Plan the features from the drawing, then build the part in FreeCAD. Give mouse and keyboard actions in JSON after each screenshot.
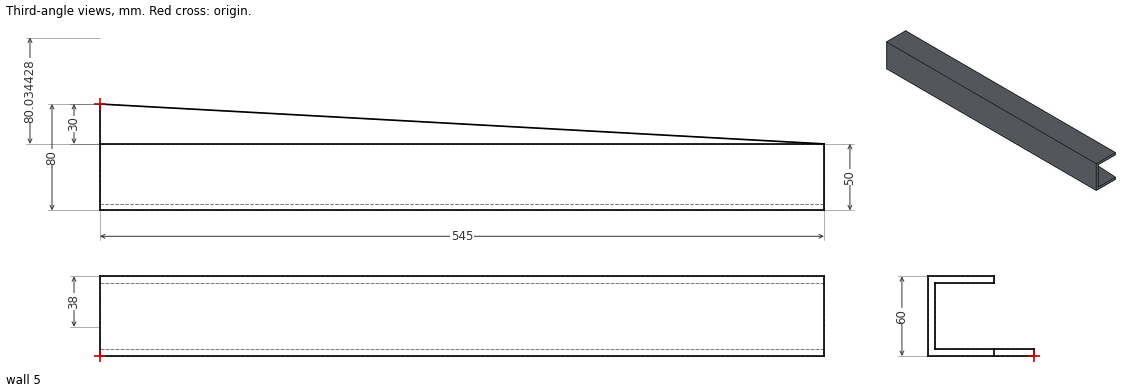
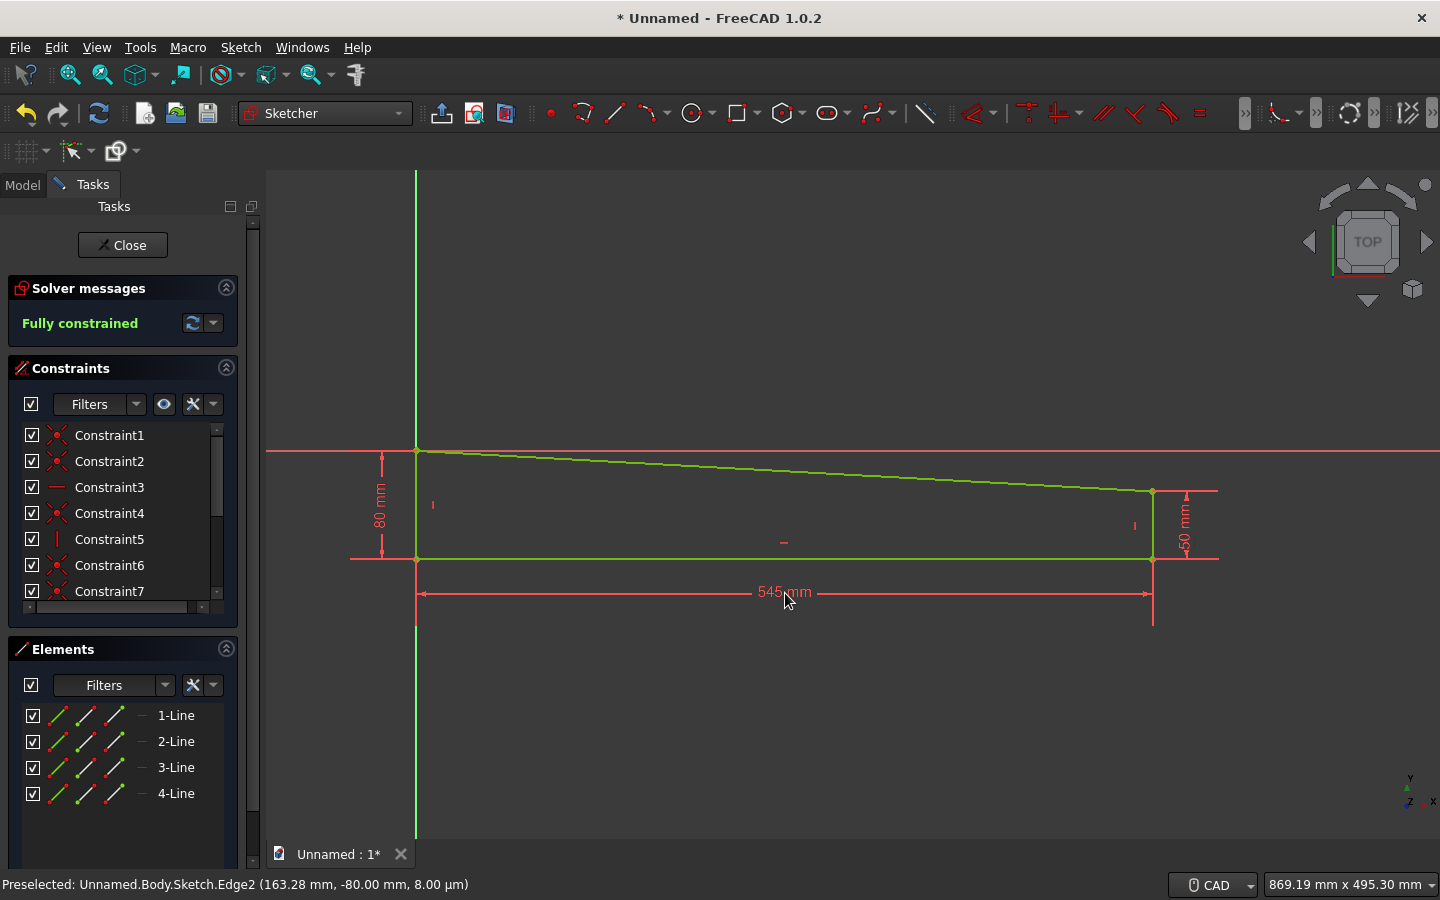
{"action": "left_click", "coordinate": [123, 245]}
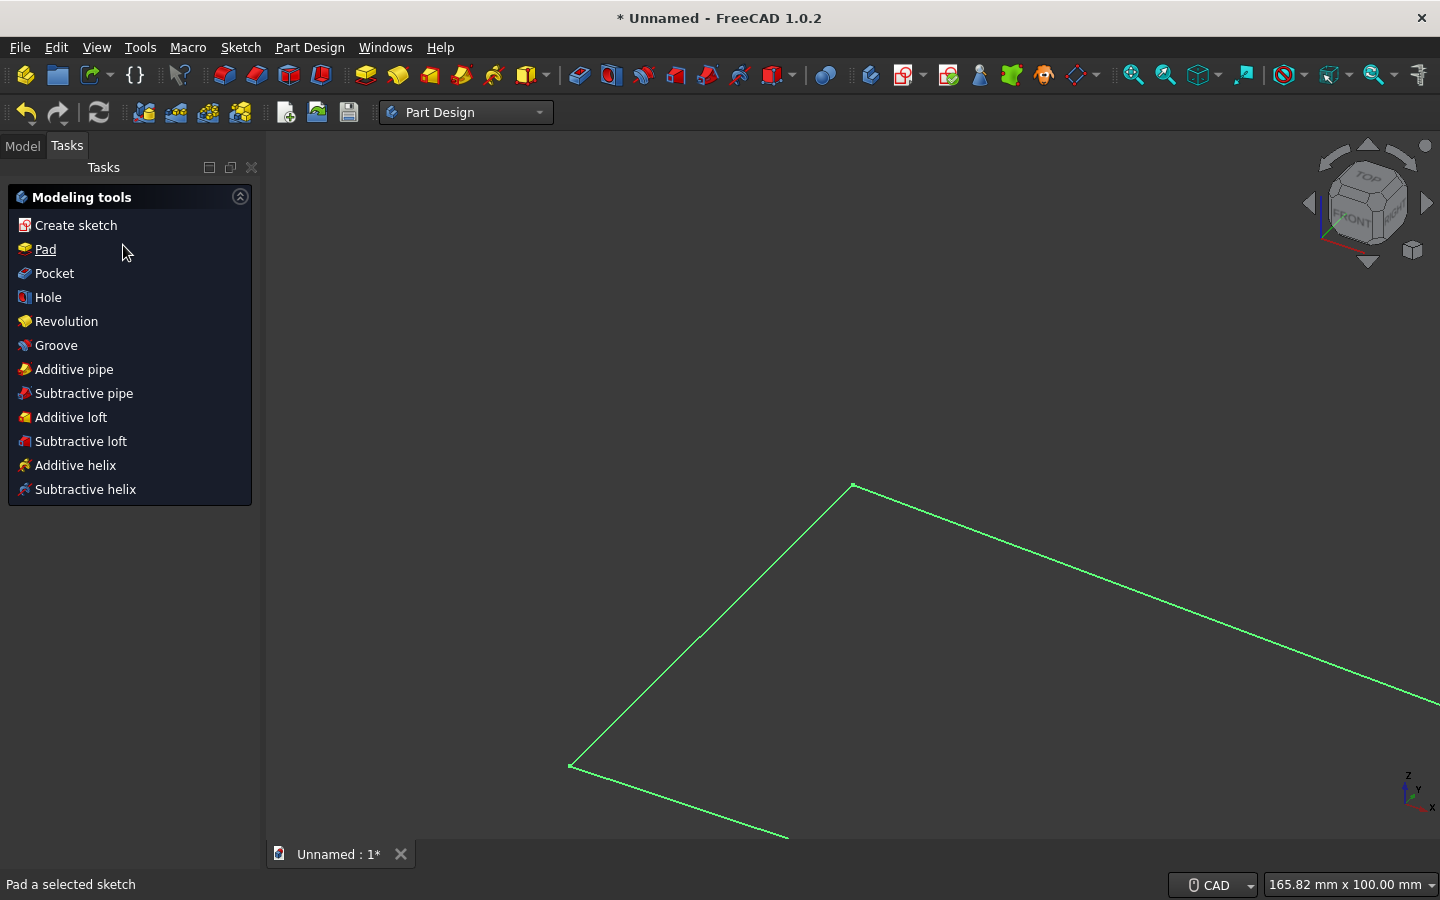
{"action": "left_click", "coordinate": [366, 76]}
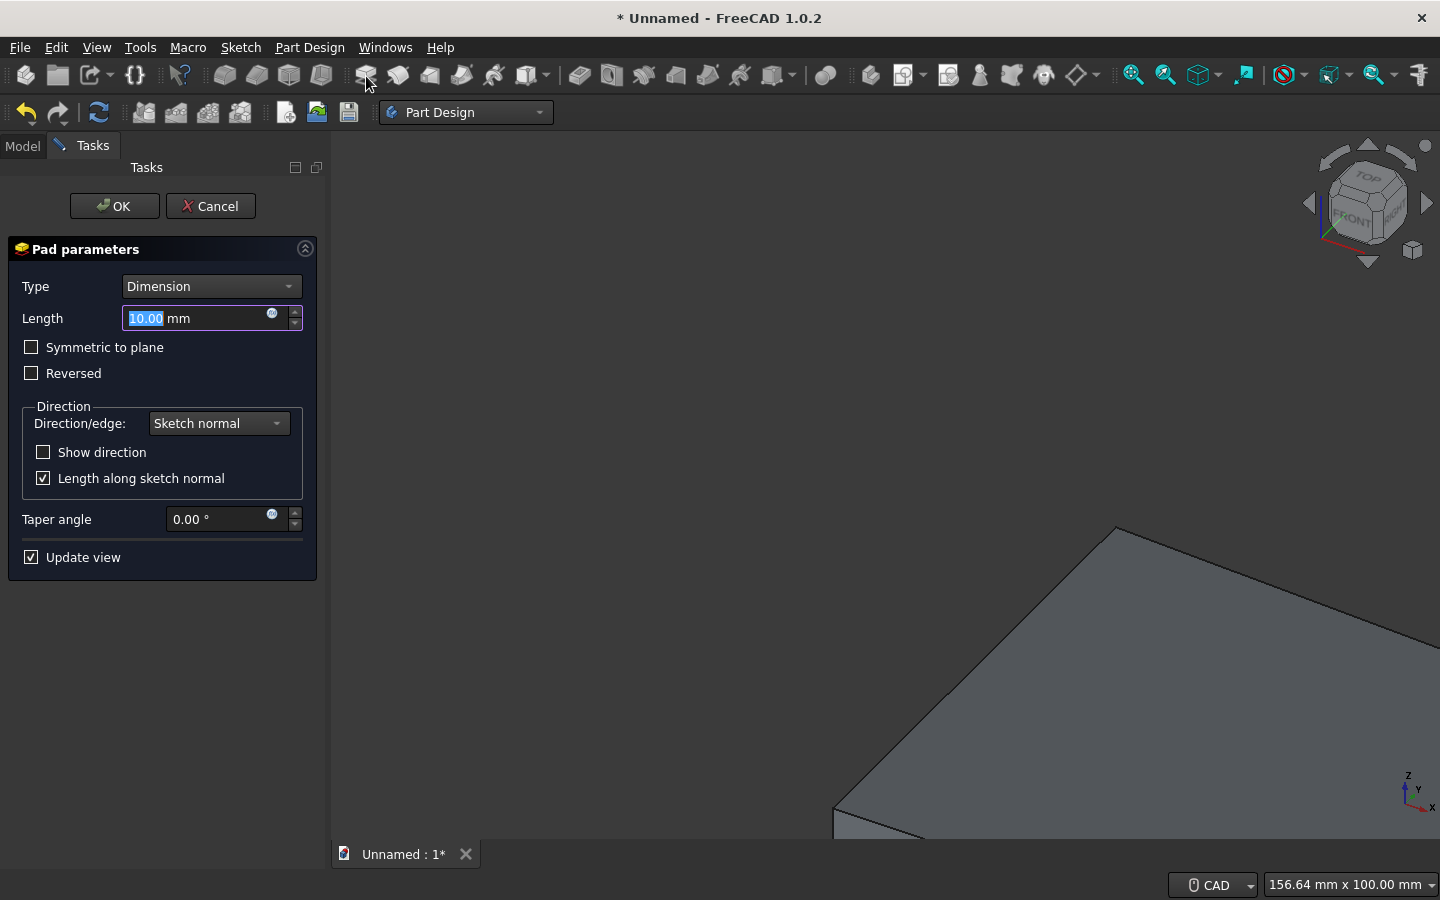
{"action": "type", "text": "60"}
{"action": "key", "text": "Tab"}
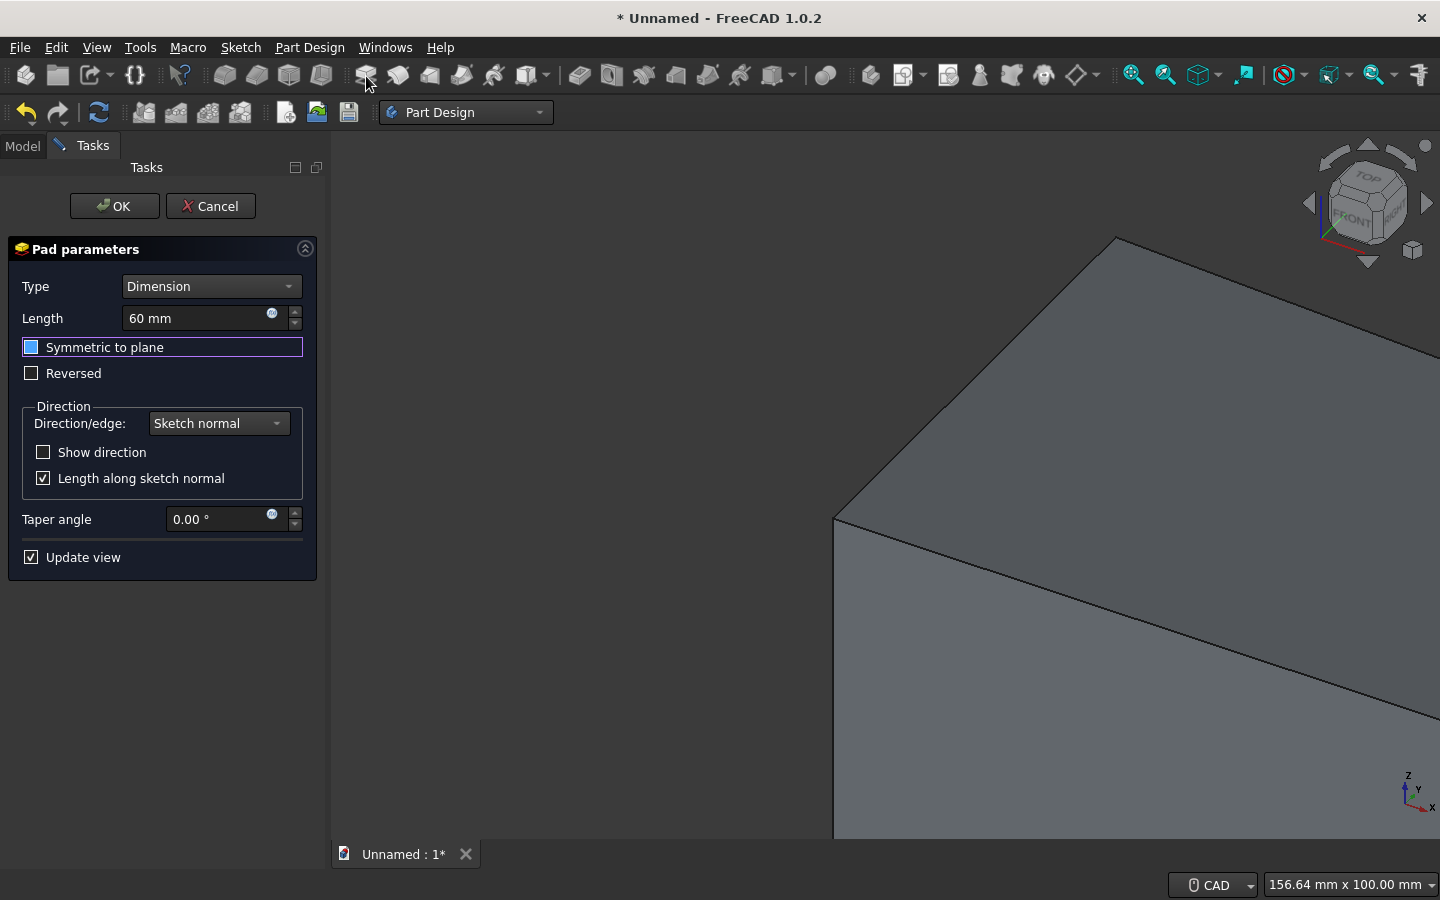
{"action": "left_click", "coordinate": [115, 206]}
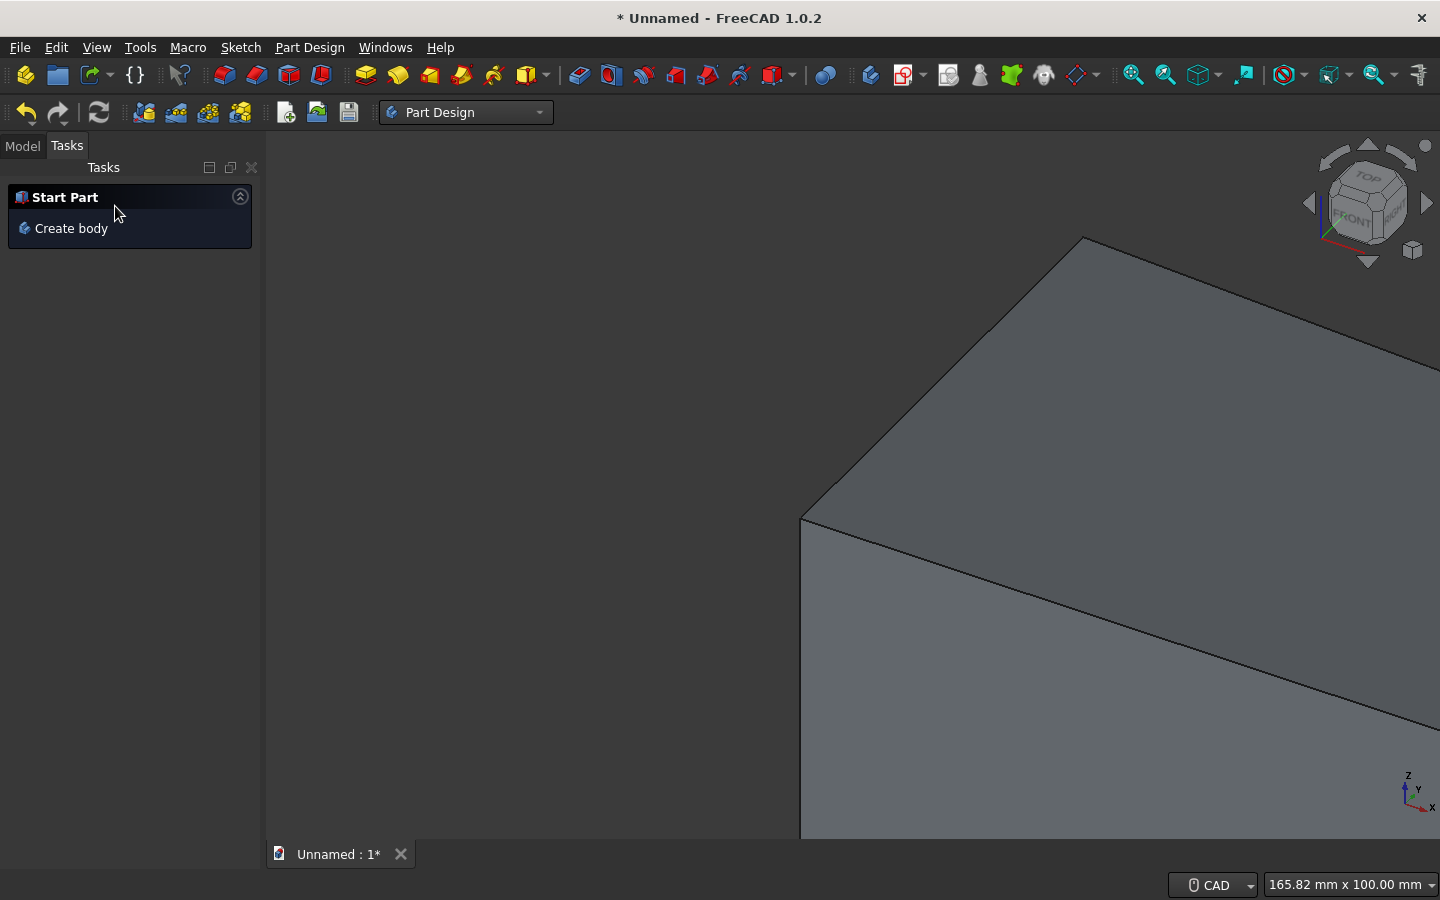
{"action": "key", "text": "v f"}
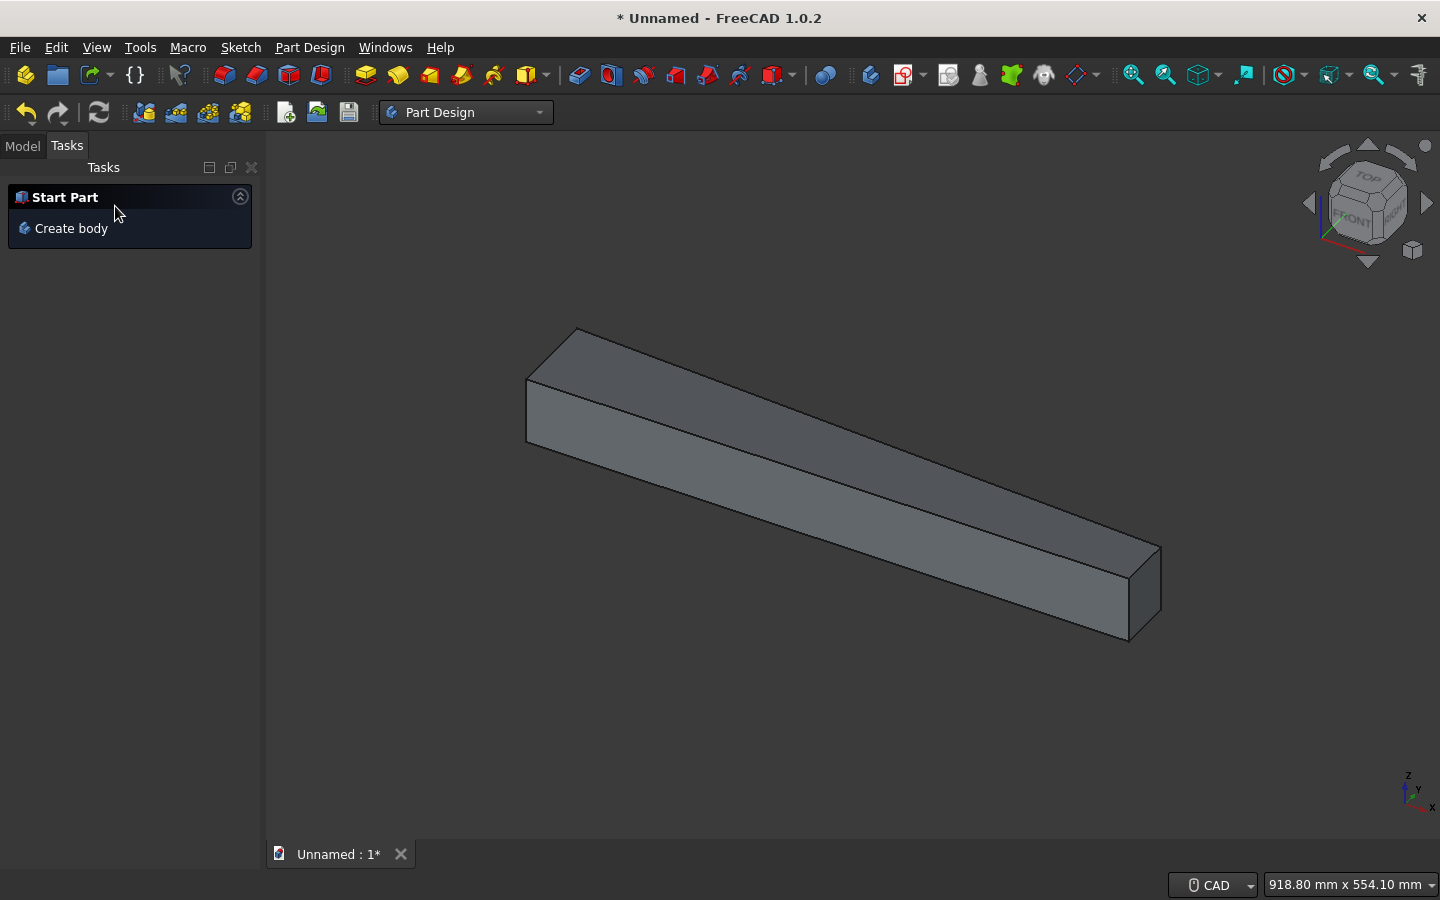
{"action": "left_click", "coordinate": [1145, 593]}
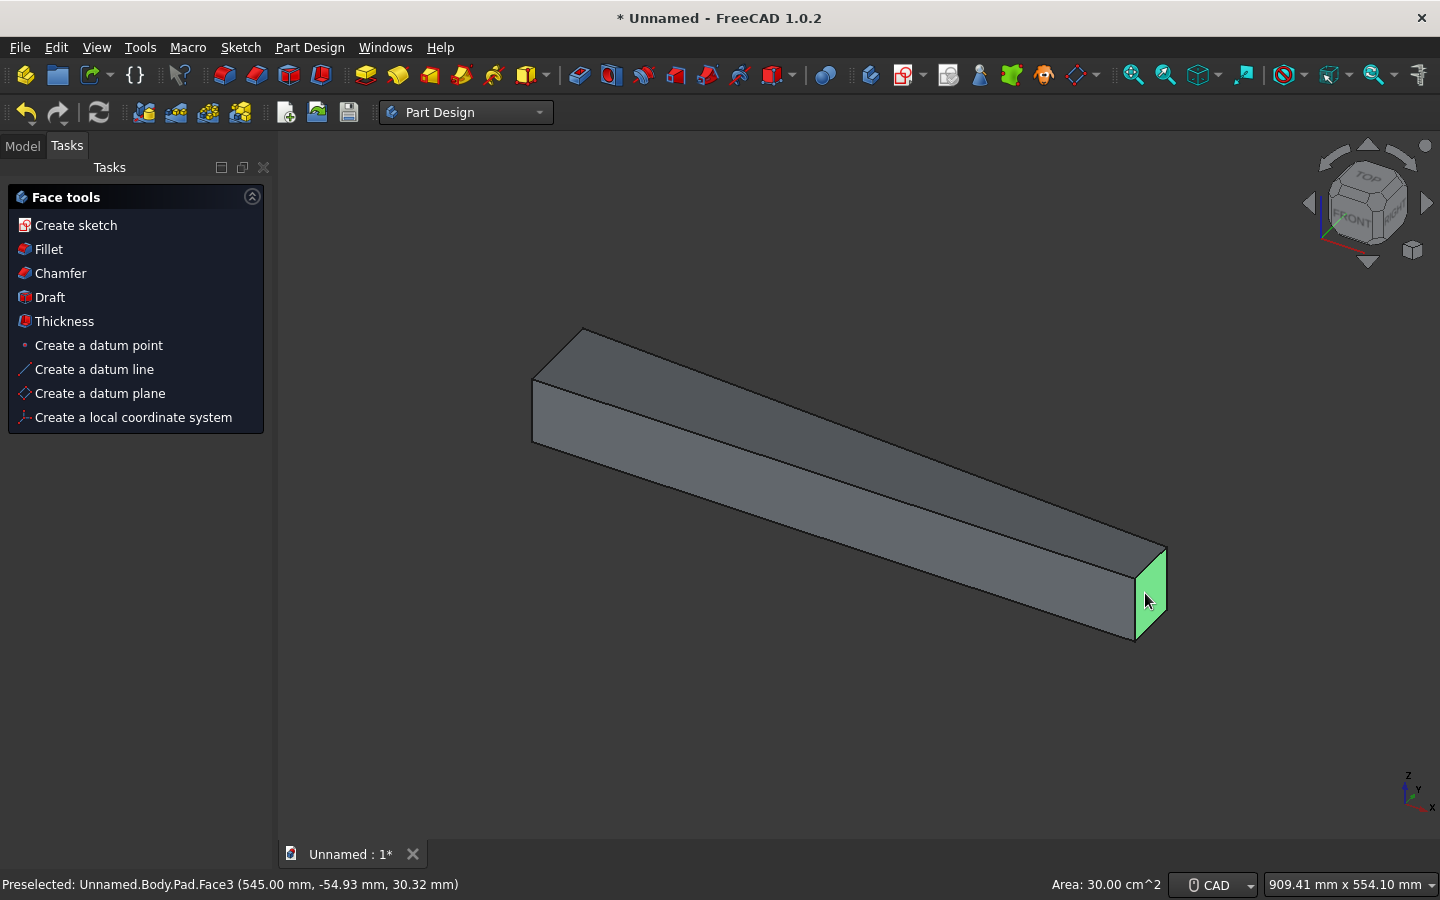
{"action": "key", "text": "0"}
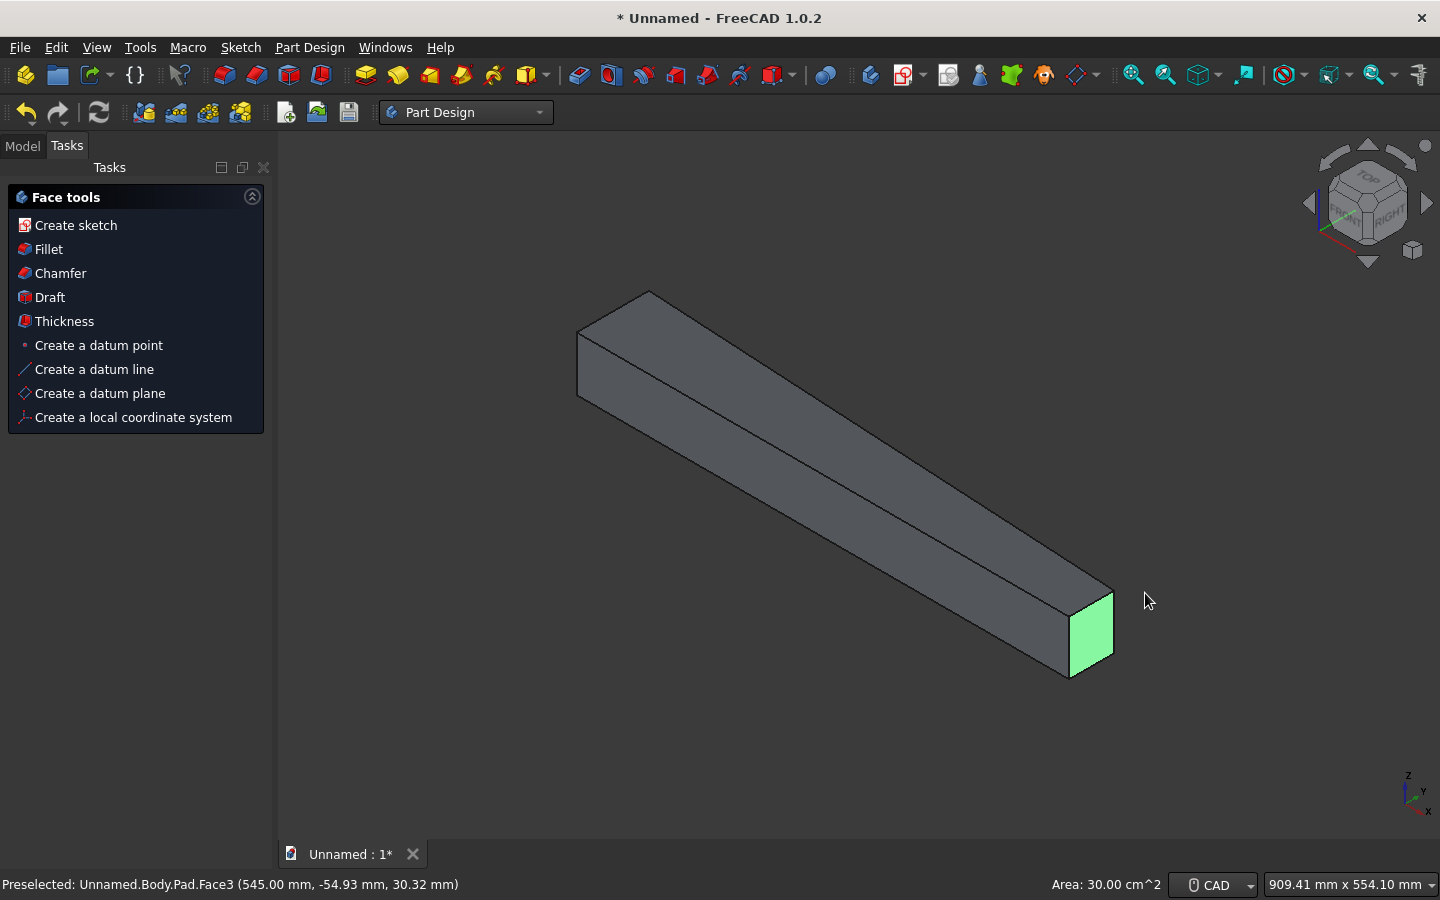
{"action": "key", "text": "2"}